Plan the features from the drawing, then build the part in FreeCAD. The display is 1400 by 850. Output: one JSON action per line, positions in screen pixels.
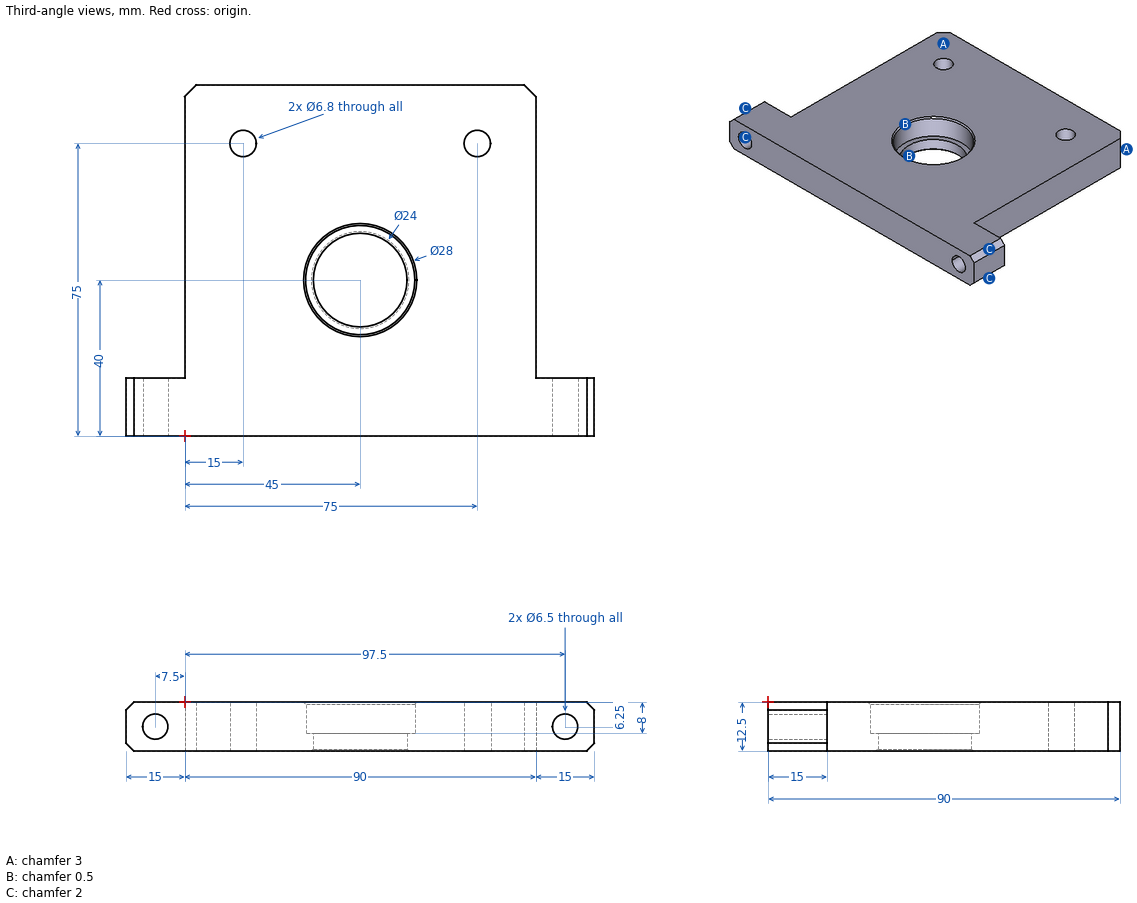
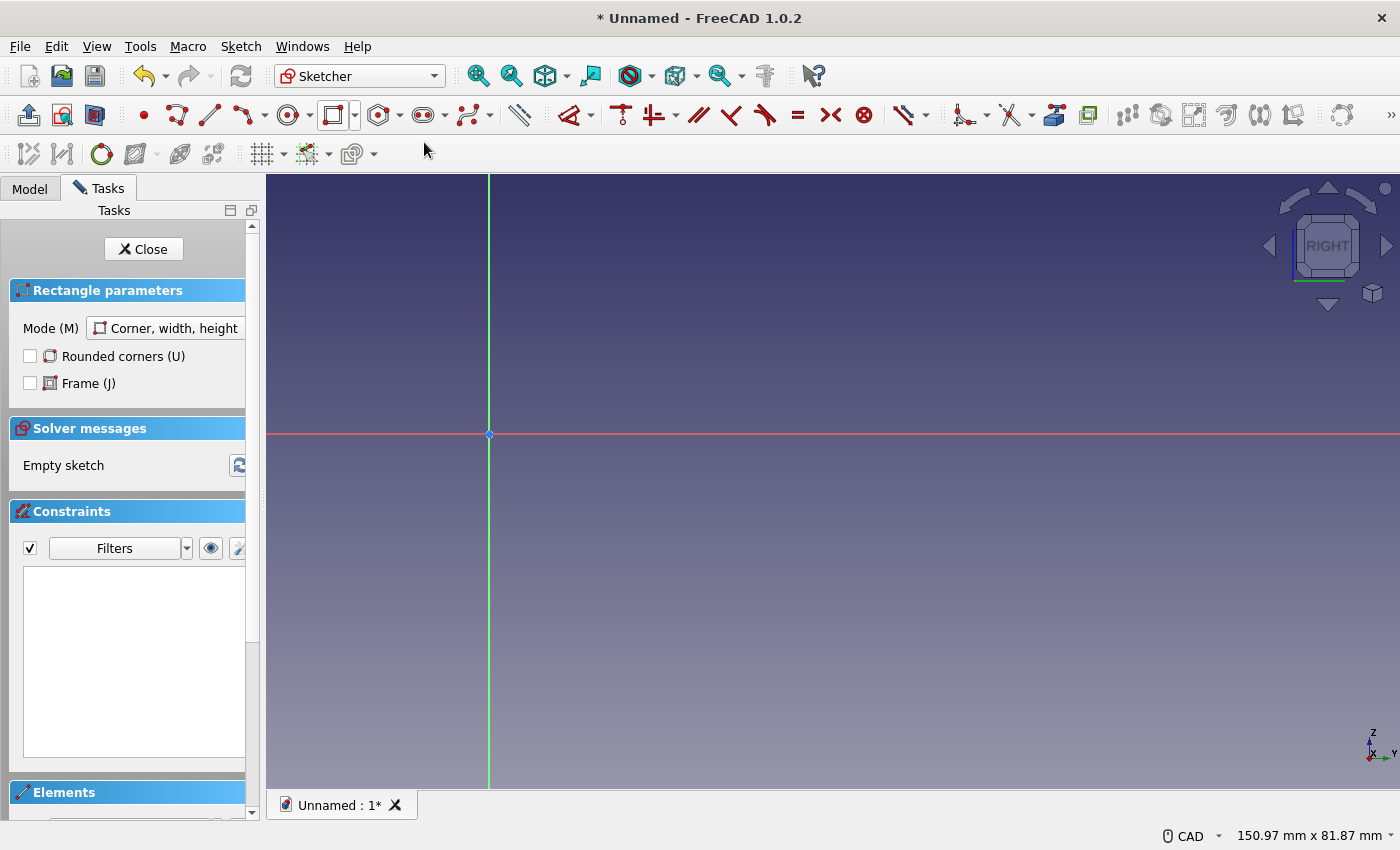
{"action": "left_click", "coordinate": [489, 434]}
{"action": "left_click", "coordinate": [1165, 528]}
{"action": "key", "text": "Escape"}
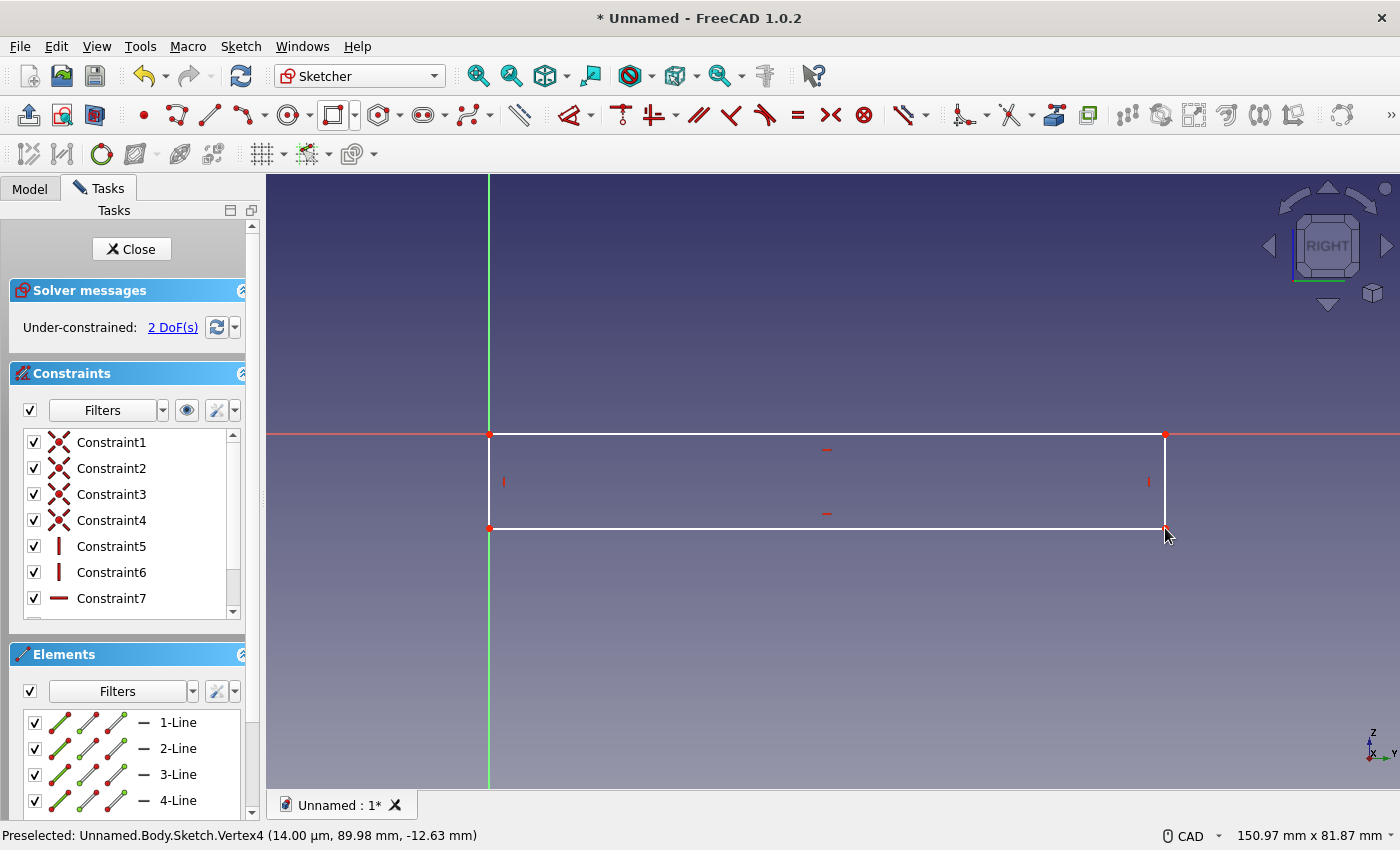
{"action": "left_click", "coordinate": [568, 116]}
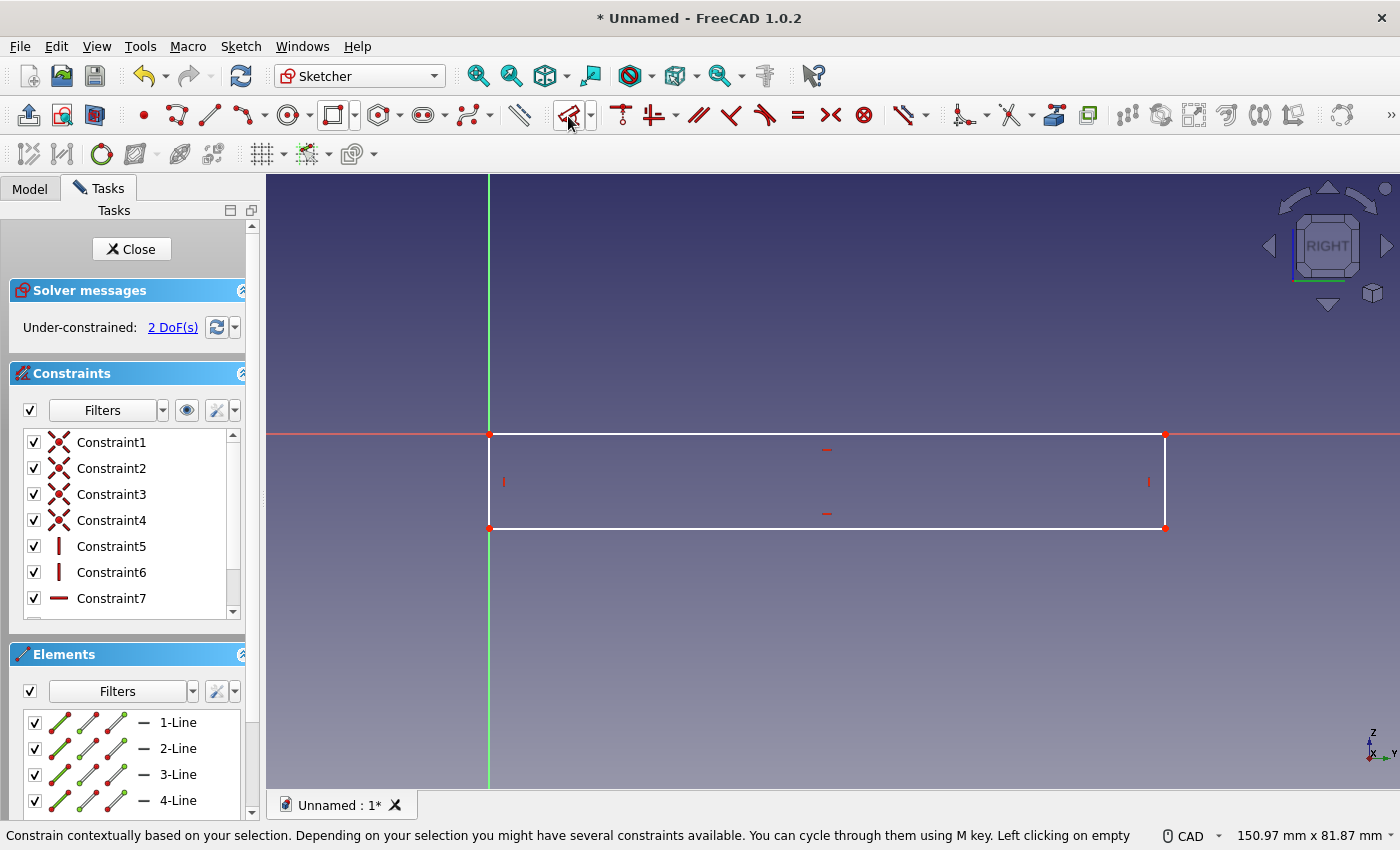
{"action": "left_click", "coordinate": [692, 529]}
{"action": "left_click", "coordinate": [827, 563]}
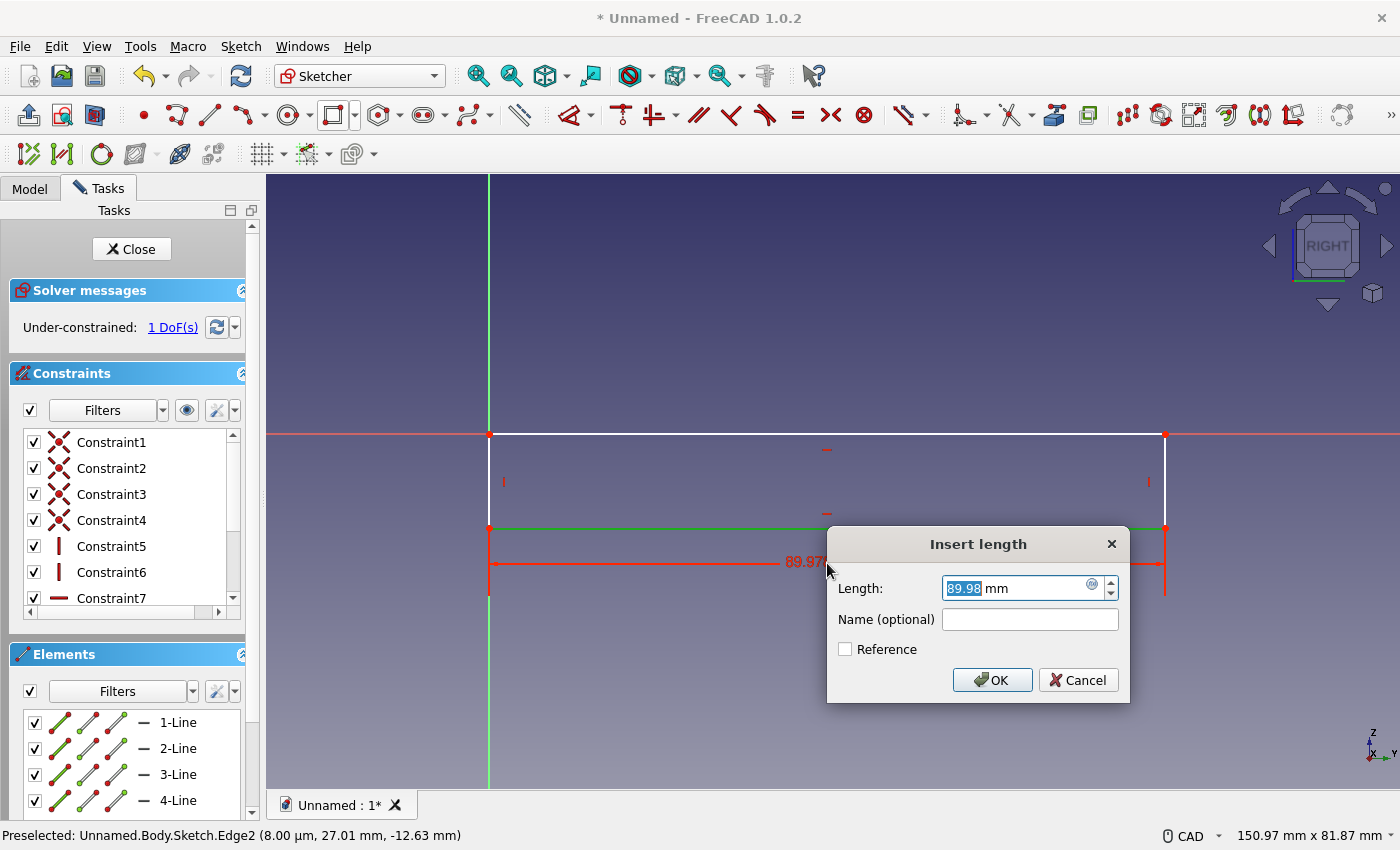
{"action": "type", "text": "90"}
{"action": "key", "text": "Return"}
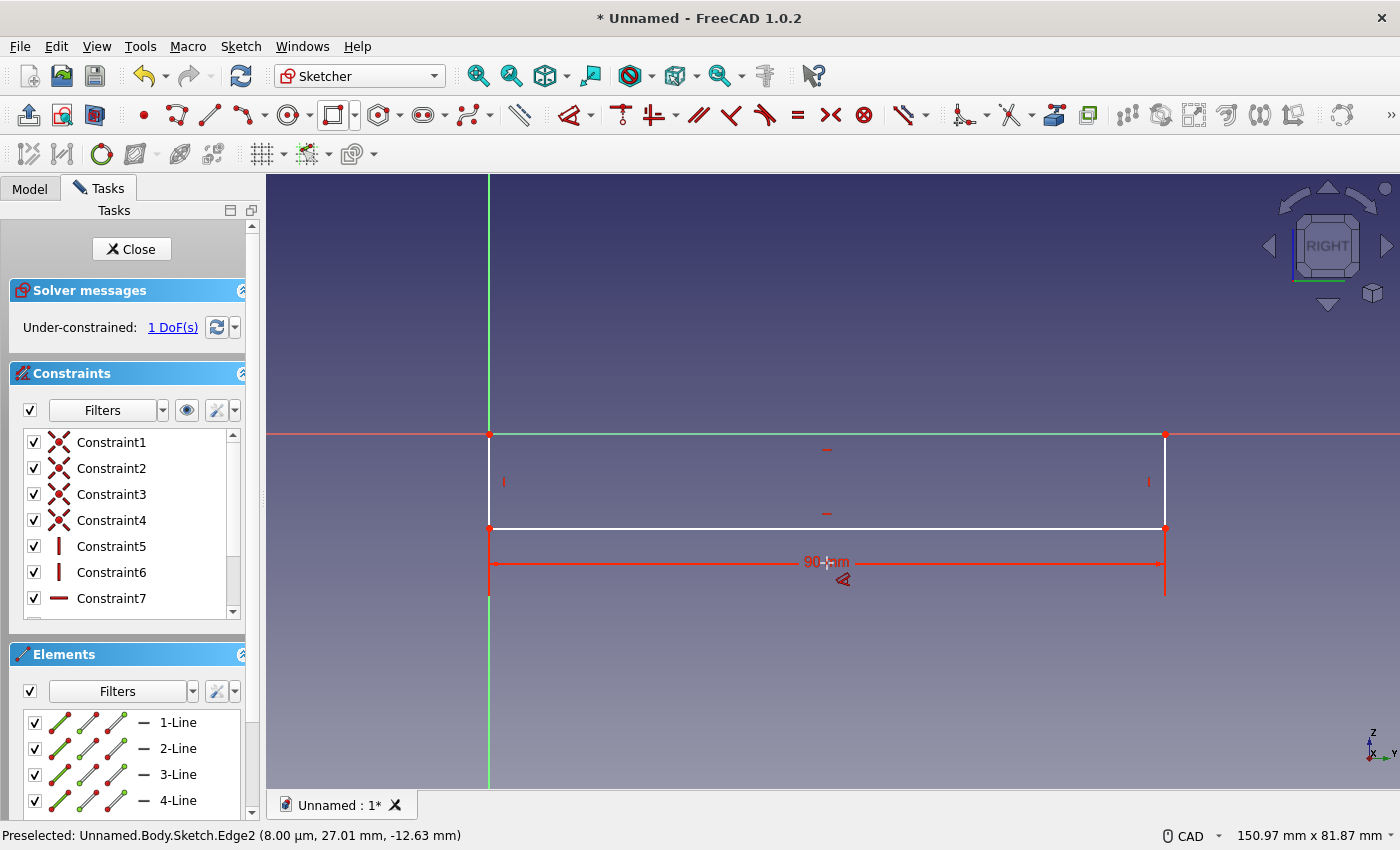
{"action": "left_click", "coordinate": [489, 463]}
{"action": "left_click", "coordinate": [455, 482]}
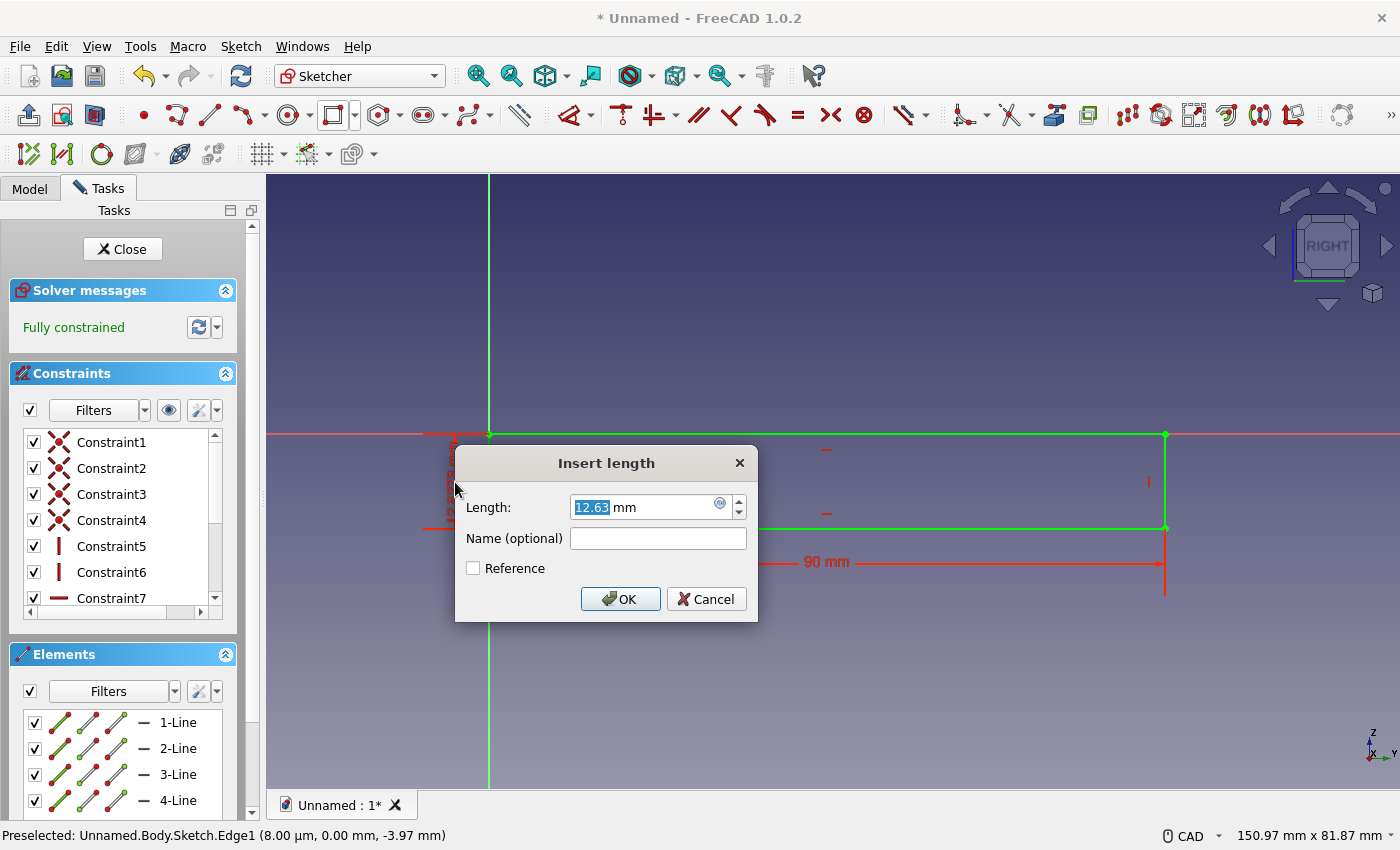
{"action": "type", "text": "12.5"}
{"action": "key", "text": "Return"}
{"action": "key", "text": "Escape"}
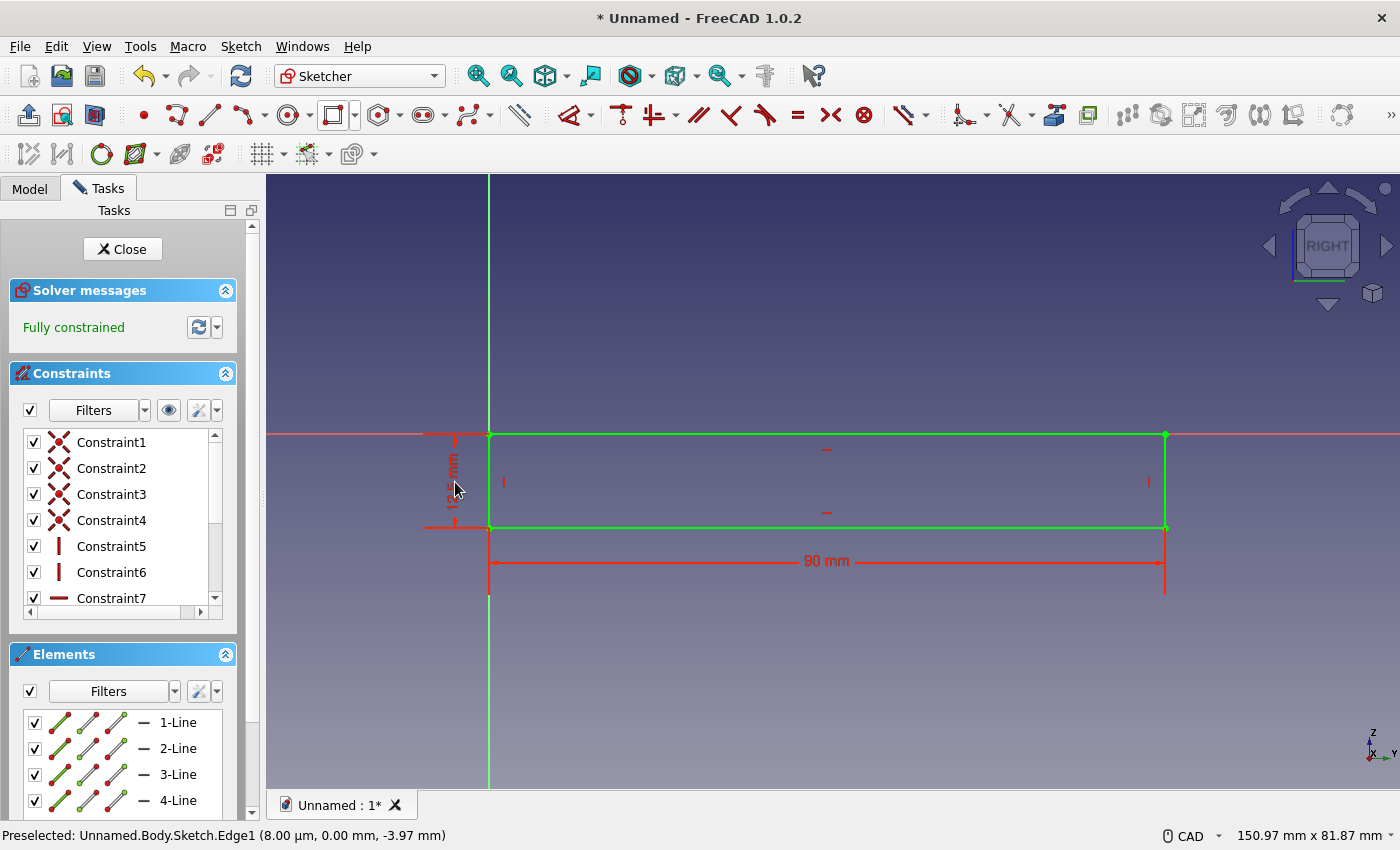
{"action": "left_click", "coordinate": [123, 249]}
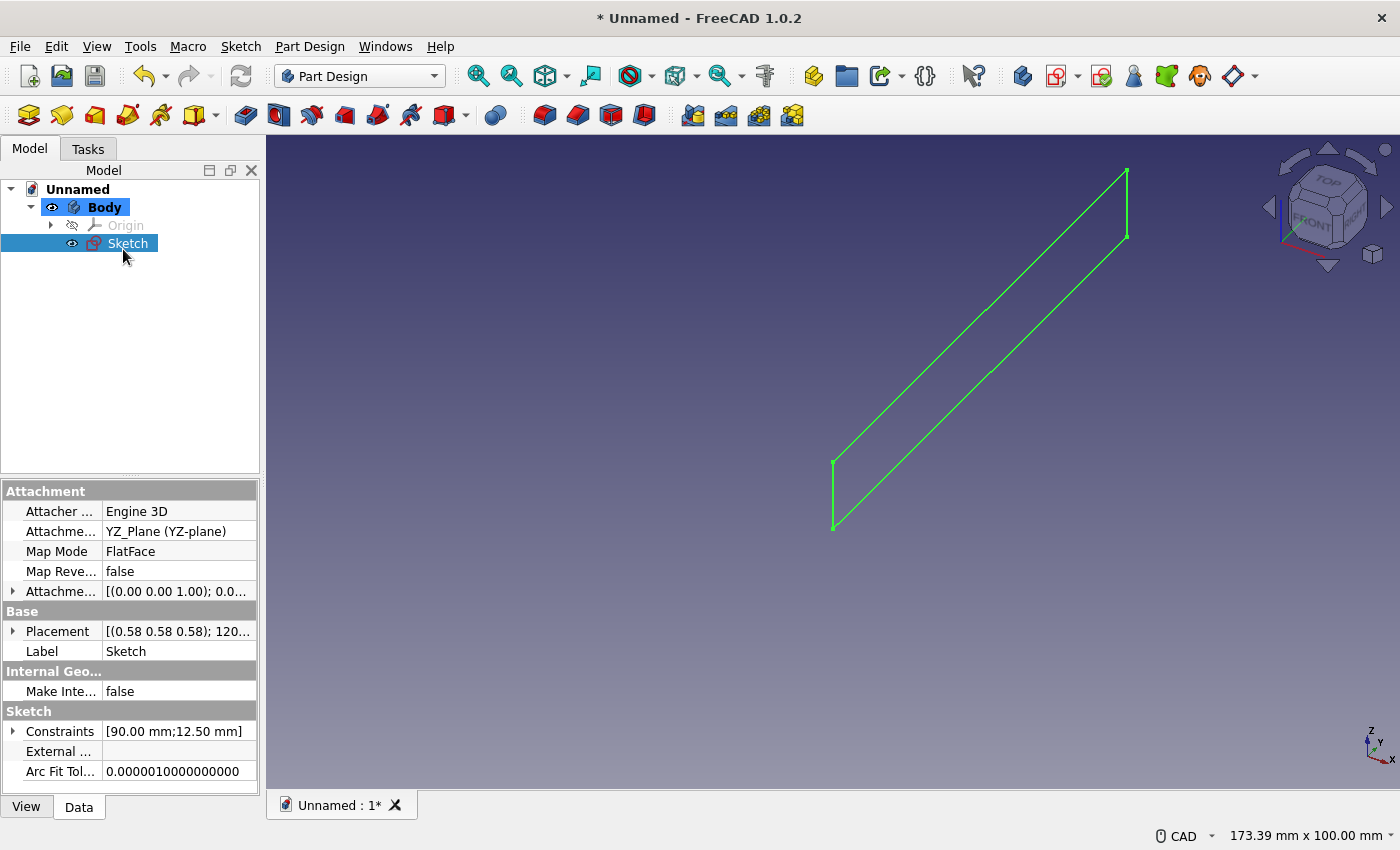
{"action": "left_click", "coordinate": [29, 116]}